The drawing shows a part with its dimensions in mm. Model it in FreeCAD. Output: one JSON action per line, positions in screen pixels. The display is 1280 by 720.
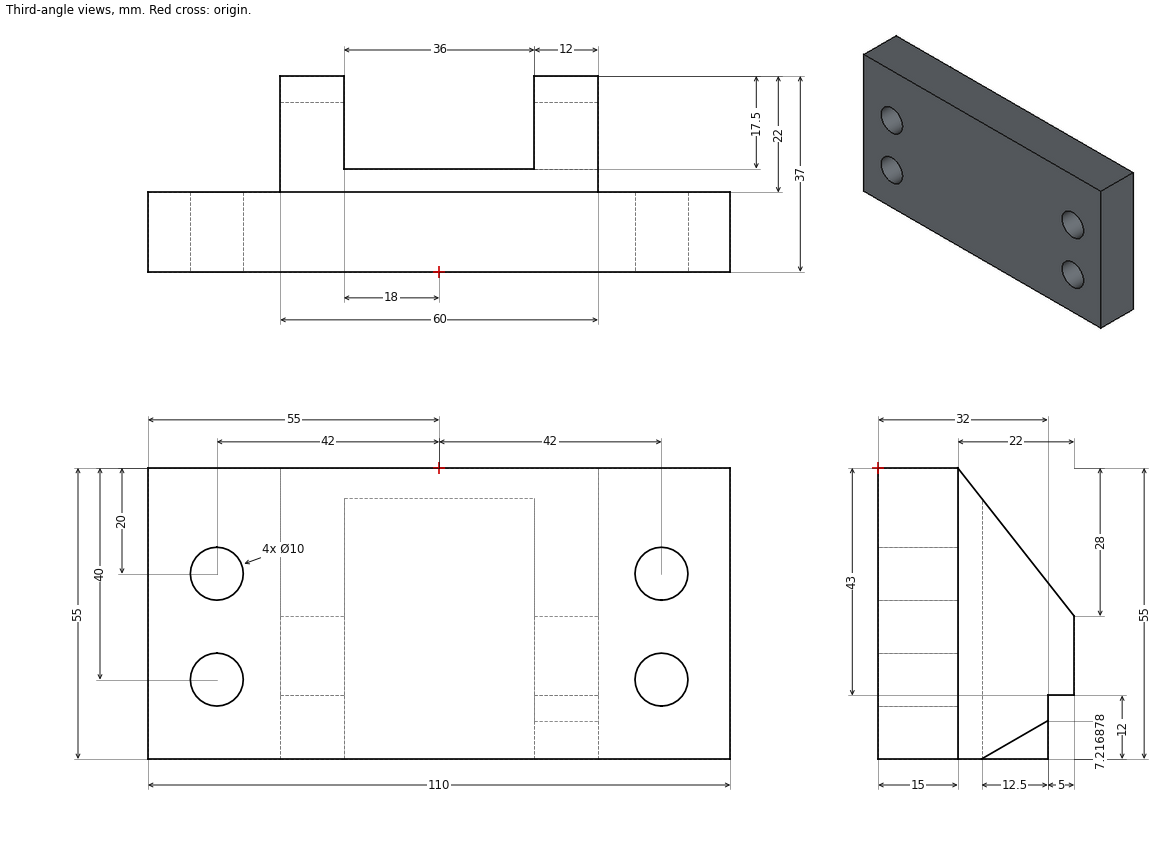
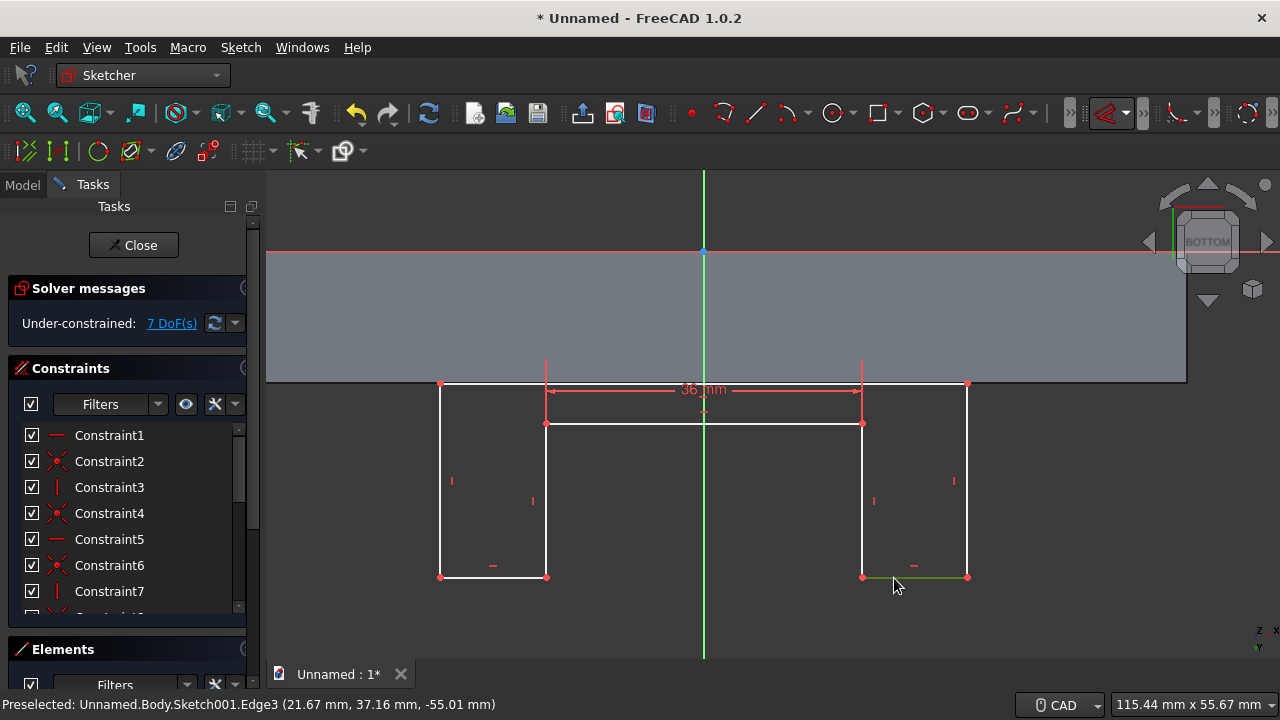
{"action": "left_click", "coordinate": [1128, 114]}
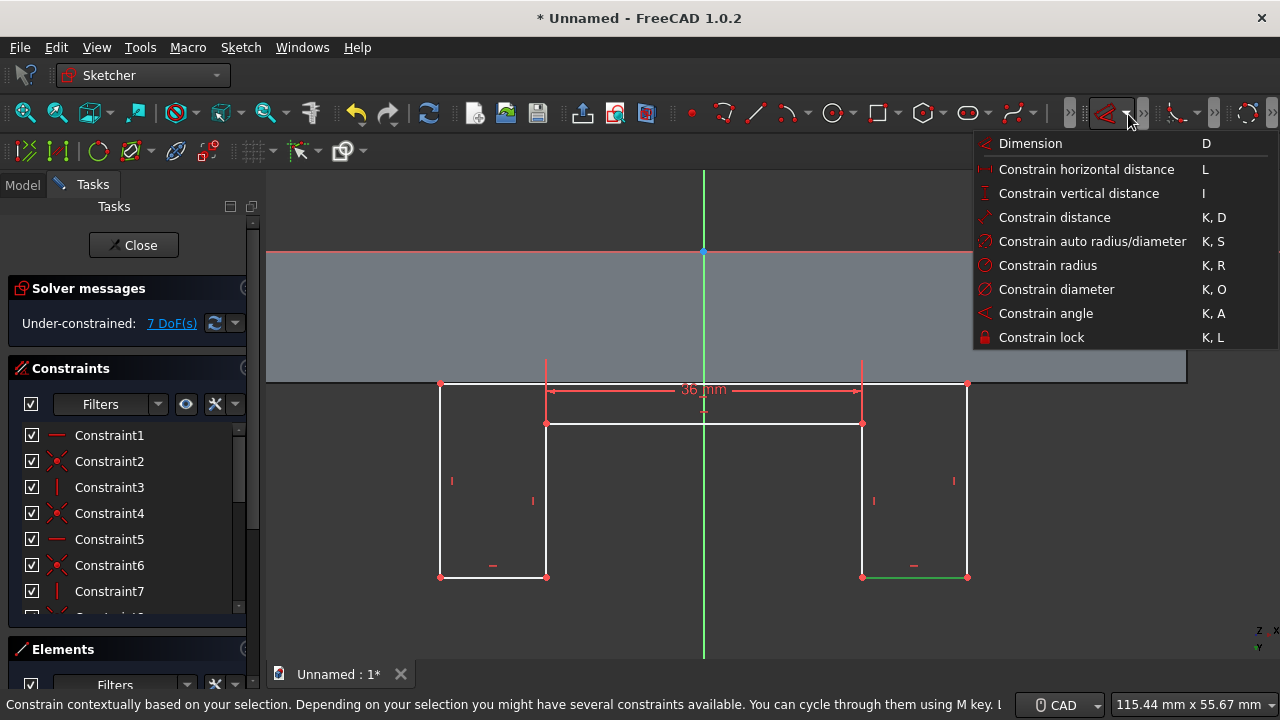
{"action": "left_click", "coordinate": [1126, 169]}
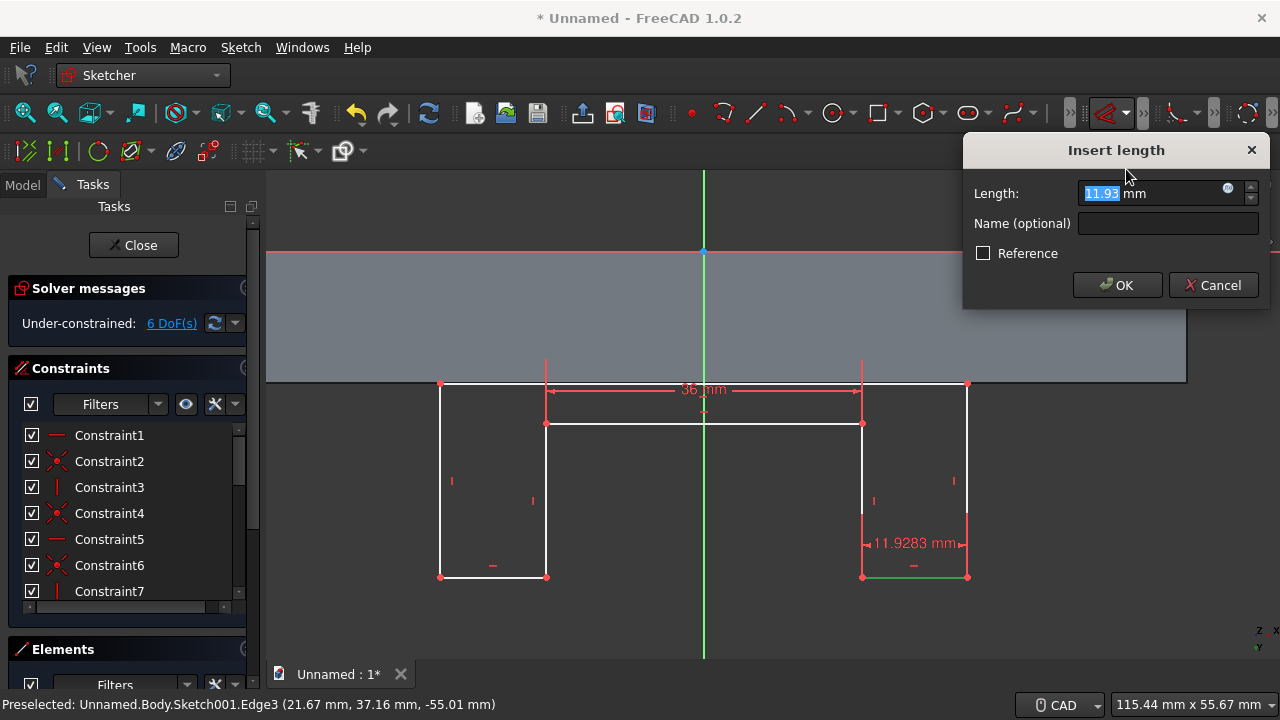
{"action": "type", "text": "12"}
{"action": "key", "text": "Return"}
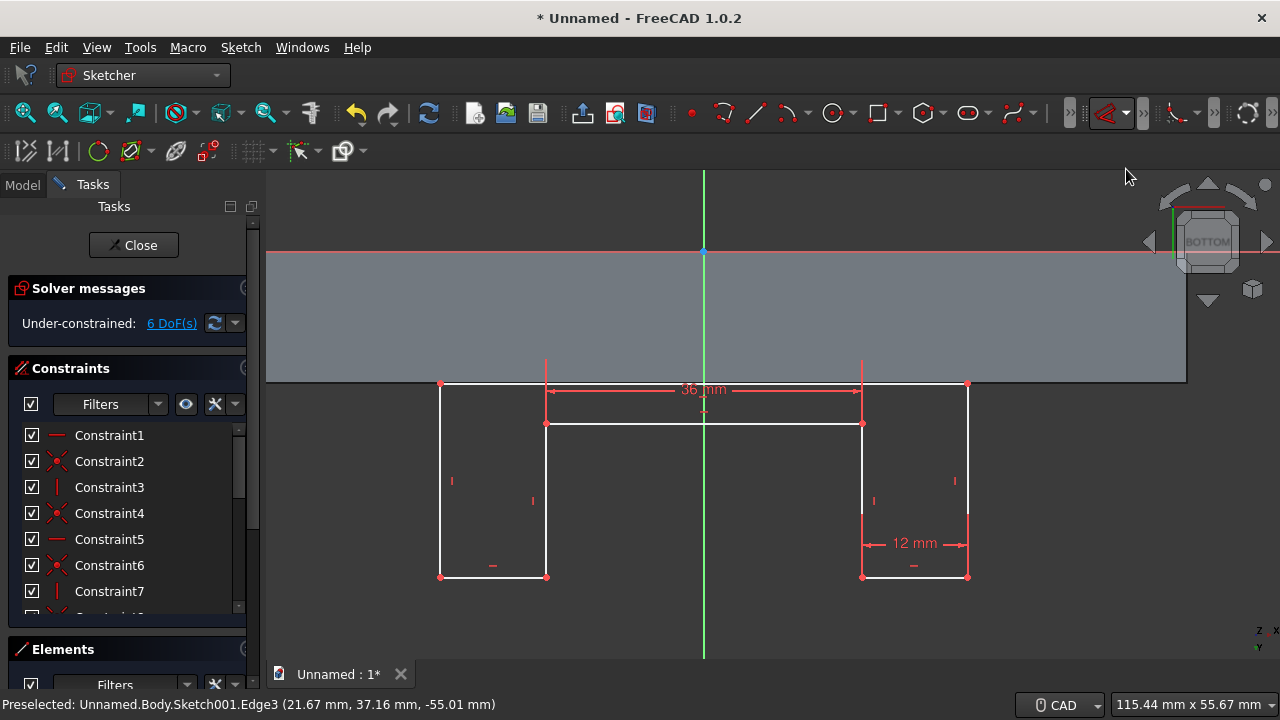
{"action": "left_click", "coordinate": [968, 520]}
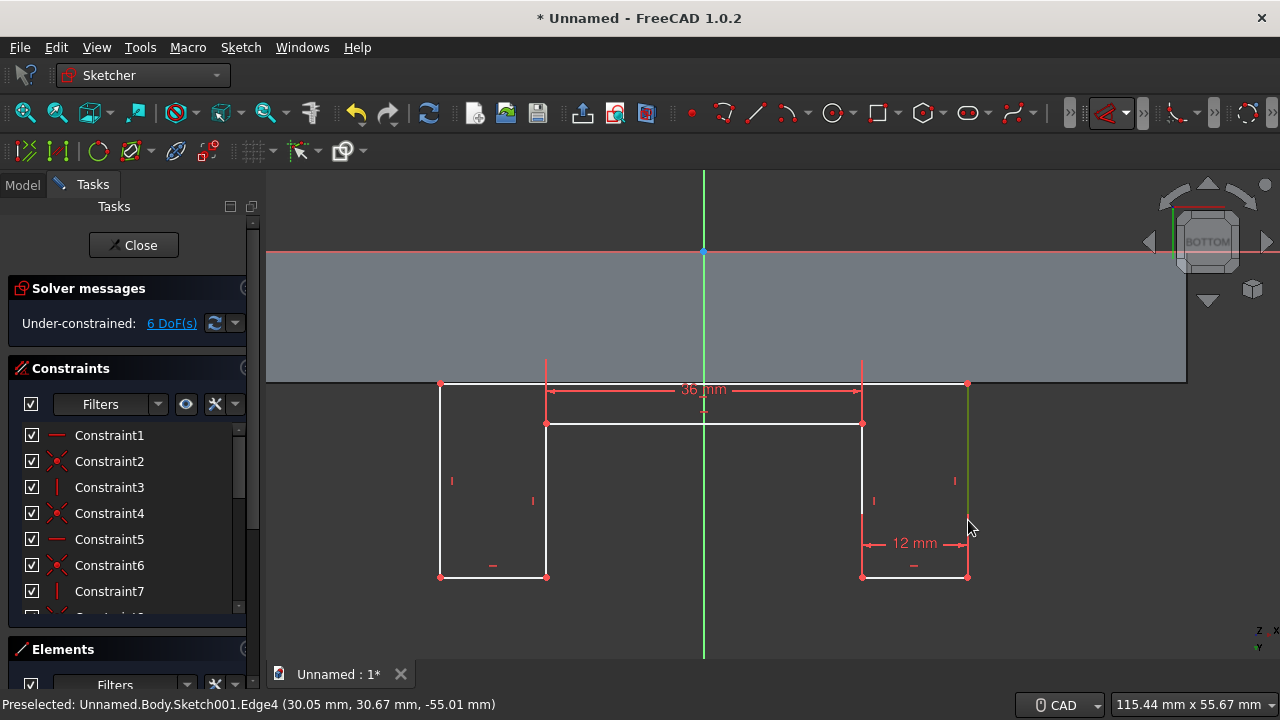
{"action": "key", "text": "i"}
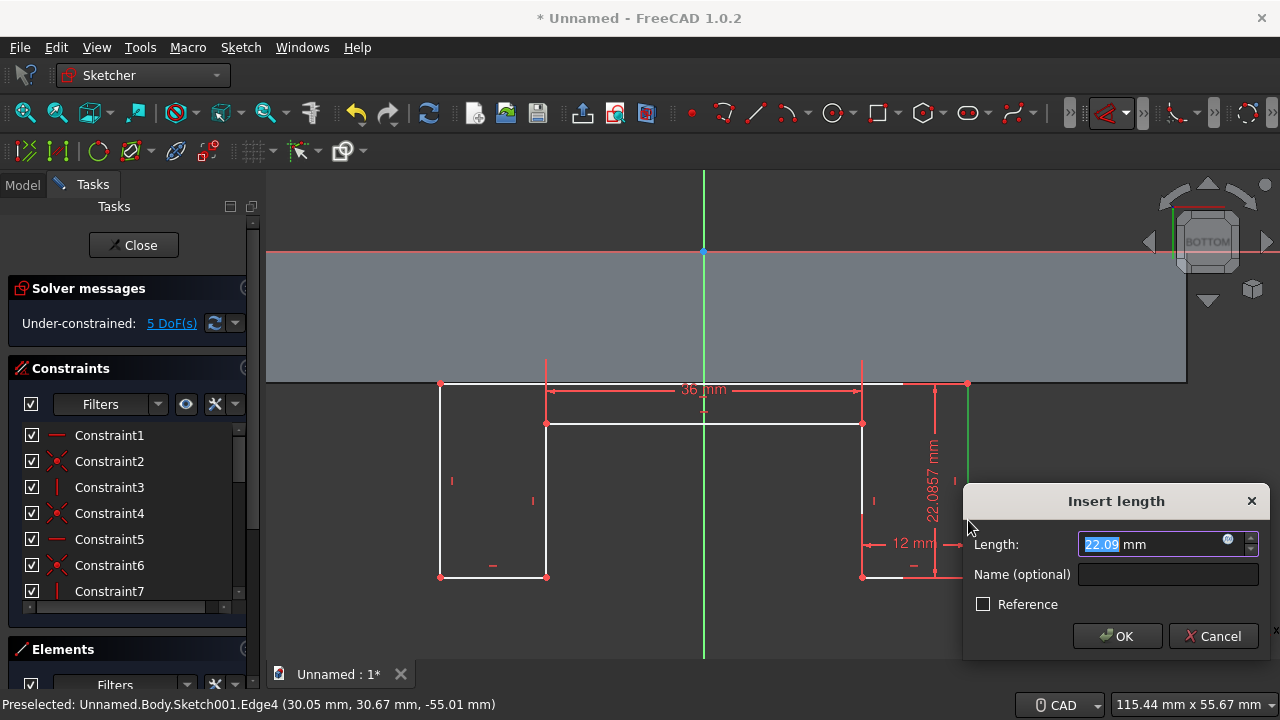
{"action": "type", "text": "22"}
{"action": "key", "text": "Return"}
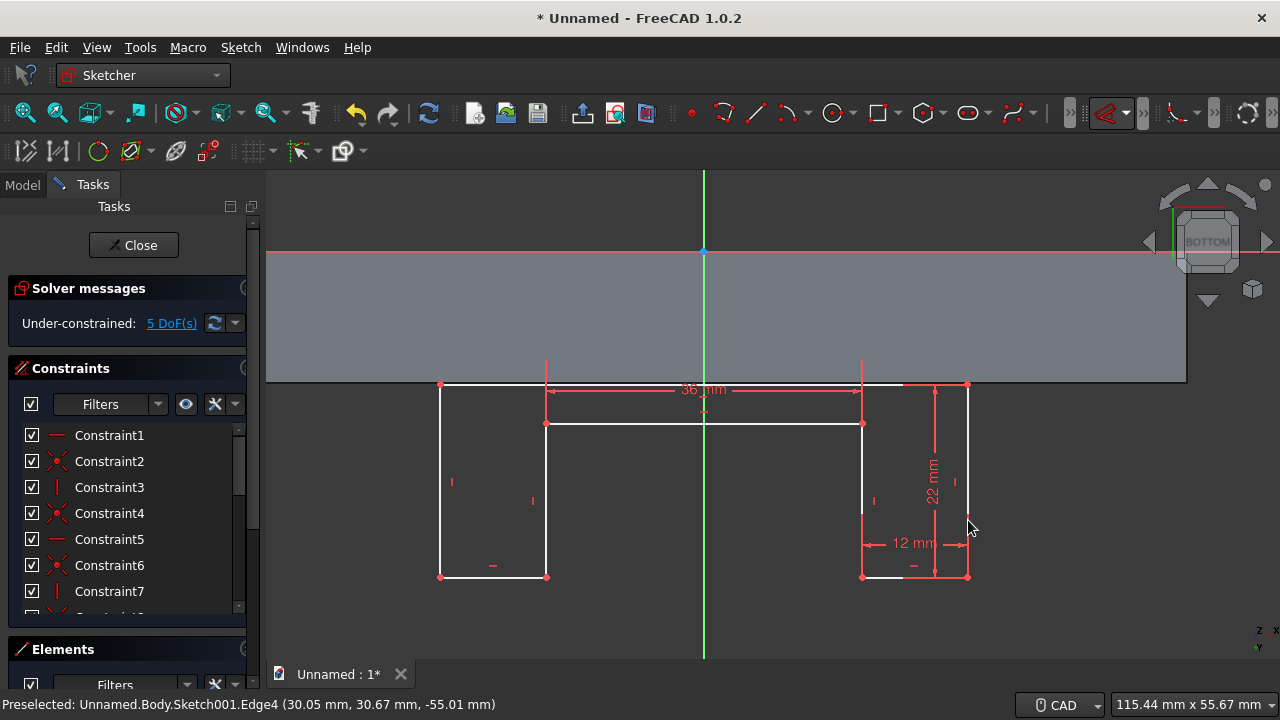
{"action": "left_click", "coordinate": [809, 385]}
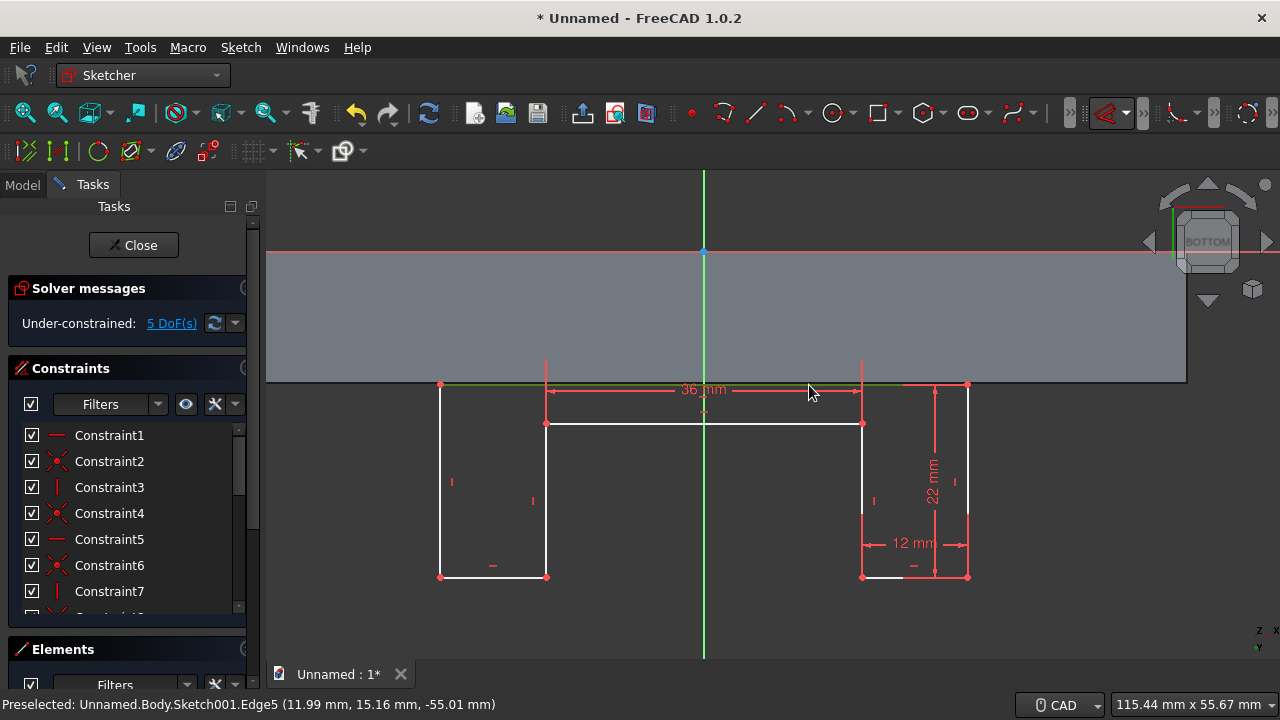
{"action": "left_click", "coordinate": [1128, 114]}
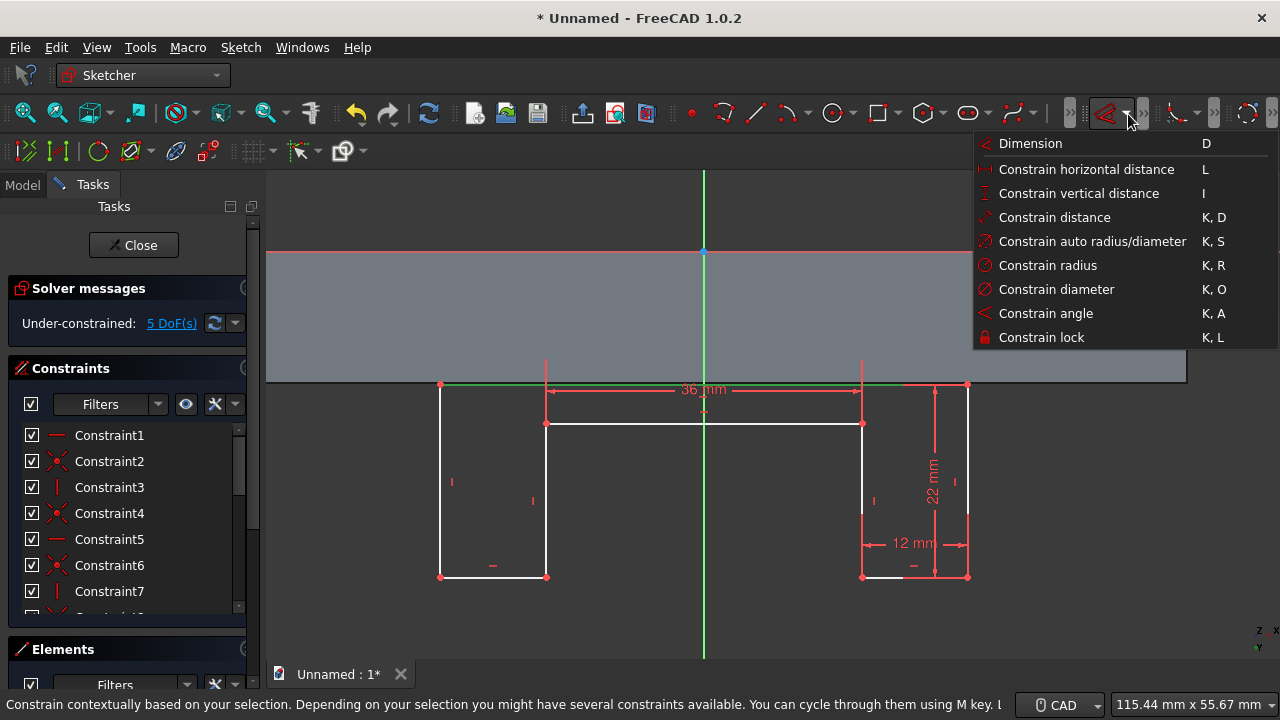
{"action": "left_click", "coordinate": [1126, 169]}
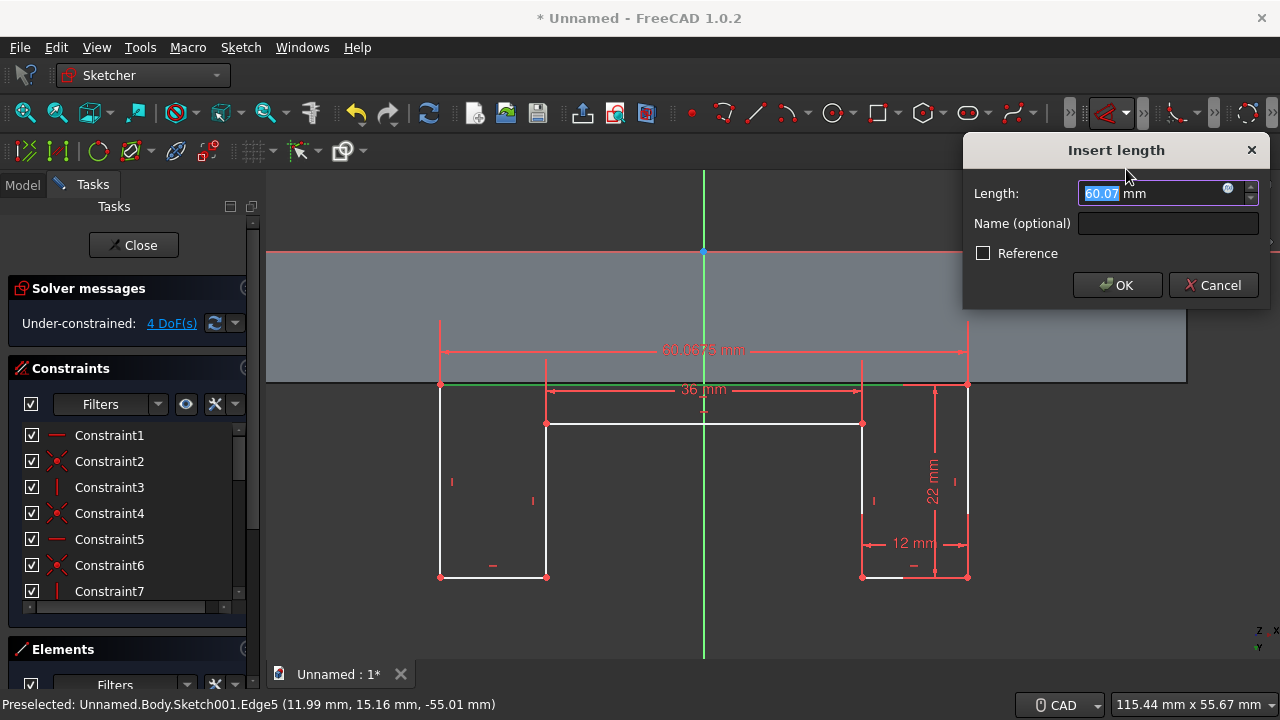
{"action": "type", "text": "60"}
{"action": "key", "text": "Return"}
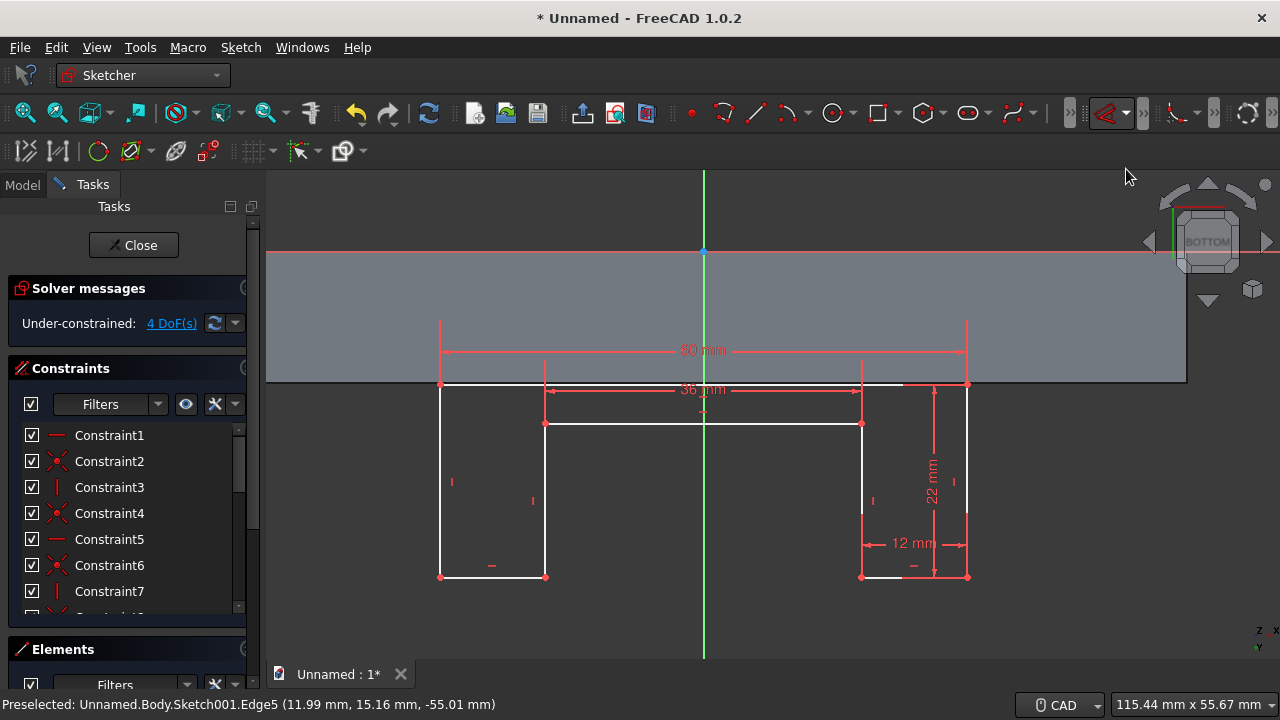
{"action": "left_click", "coordinate": [440, 443]}